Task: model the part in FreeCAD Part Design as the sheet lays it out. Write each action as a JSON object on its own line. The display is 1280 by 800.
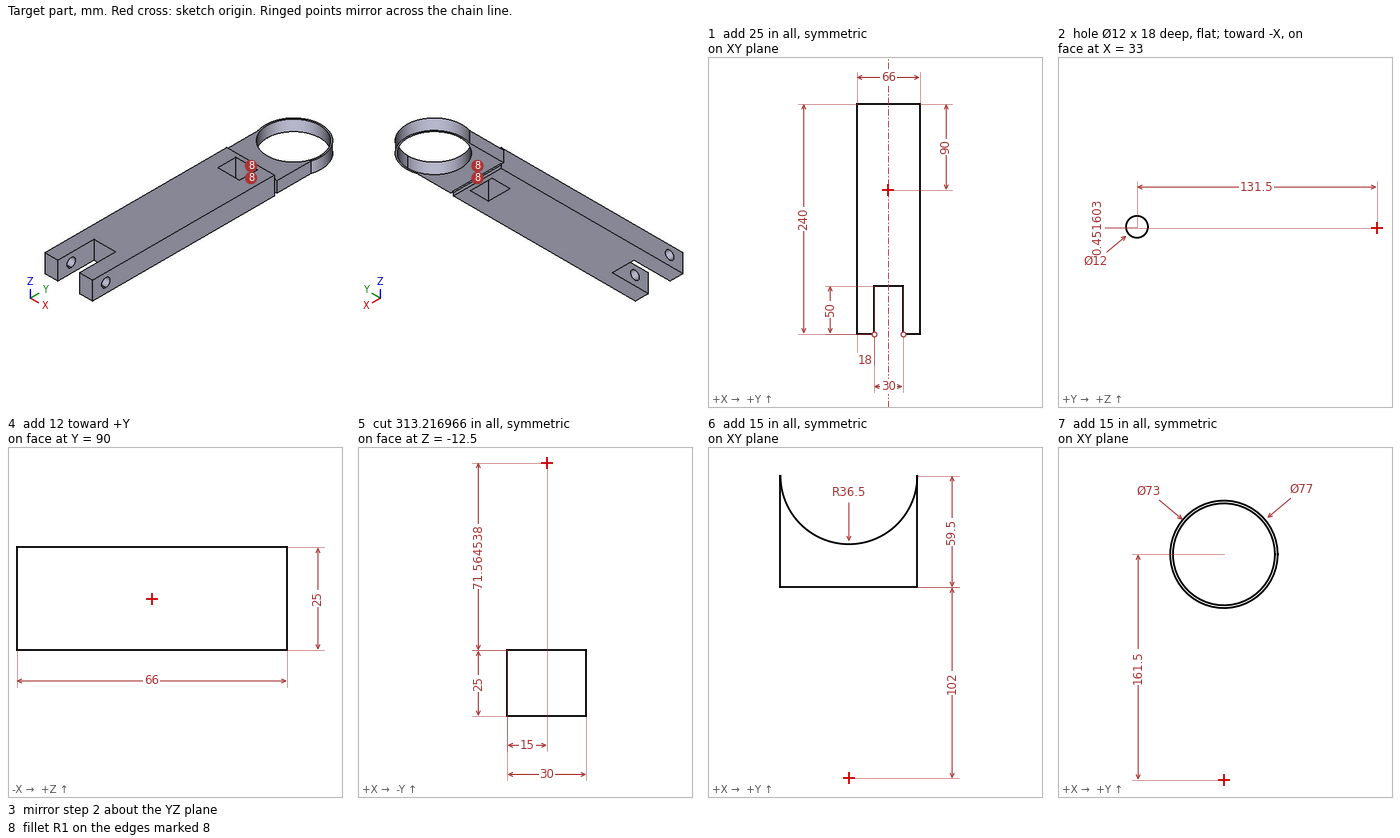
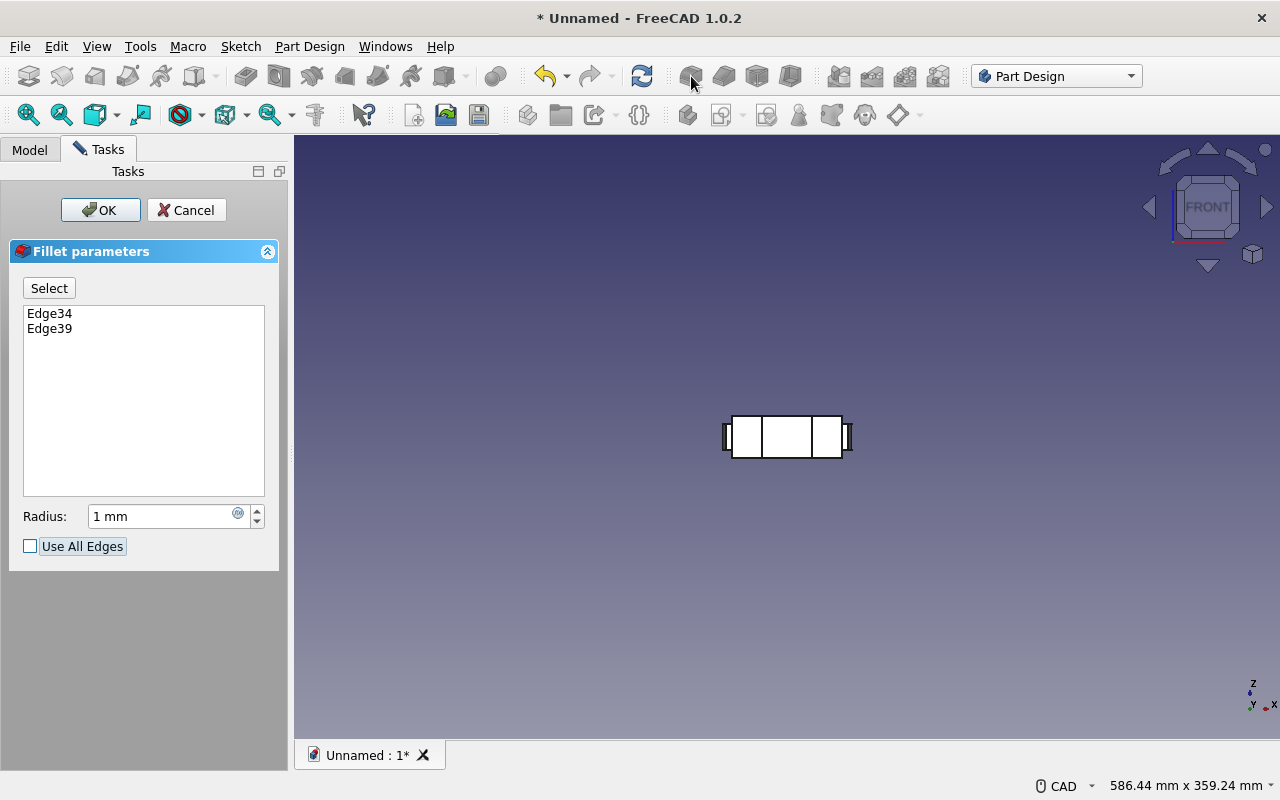
{"action": "left_click", "coordinate": [101, 210]}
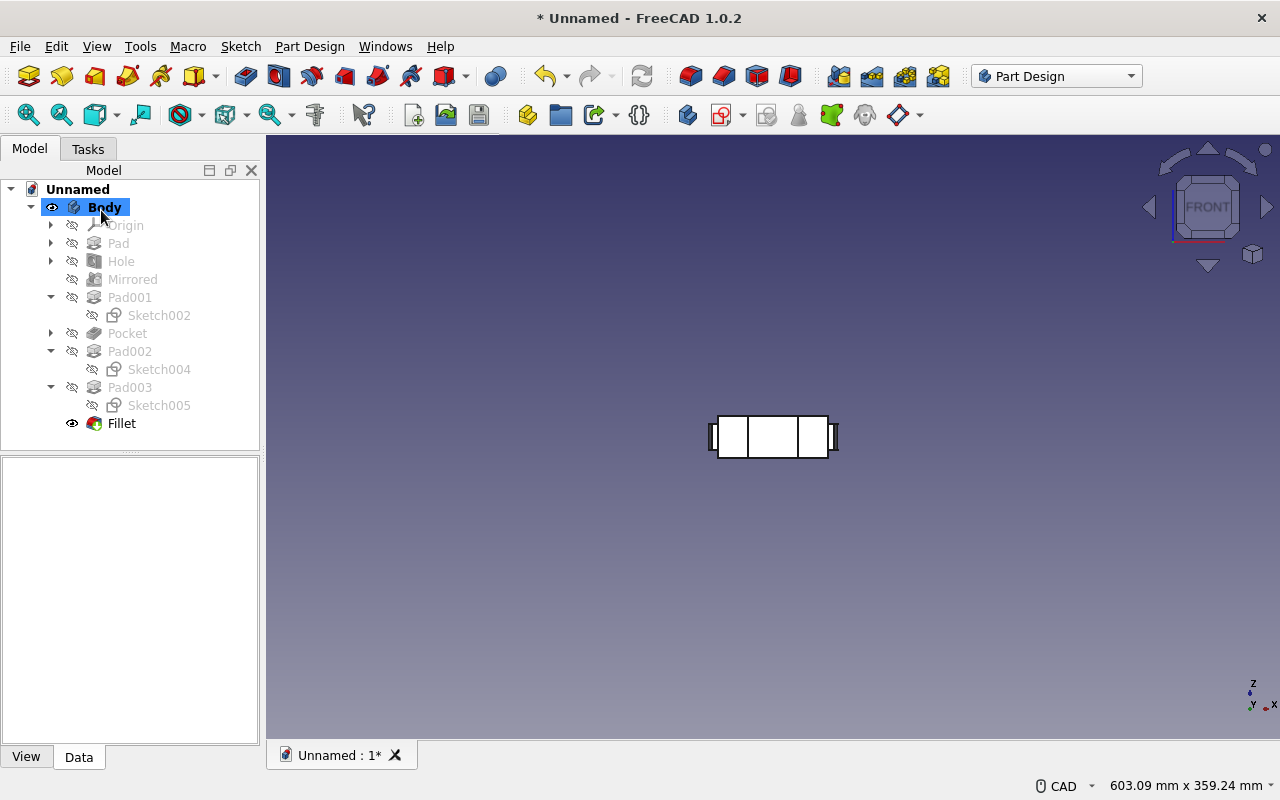
{"action": "key", "text": "0"}